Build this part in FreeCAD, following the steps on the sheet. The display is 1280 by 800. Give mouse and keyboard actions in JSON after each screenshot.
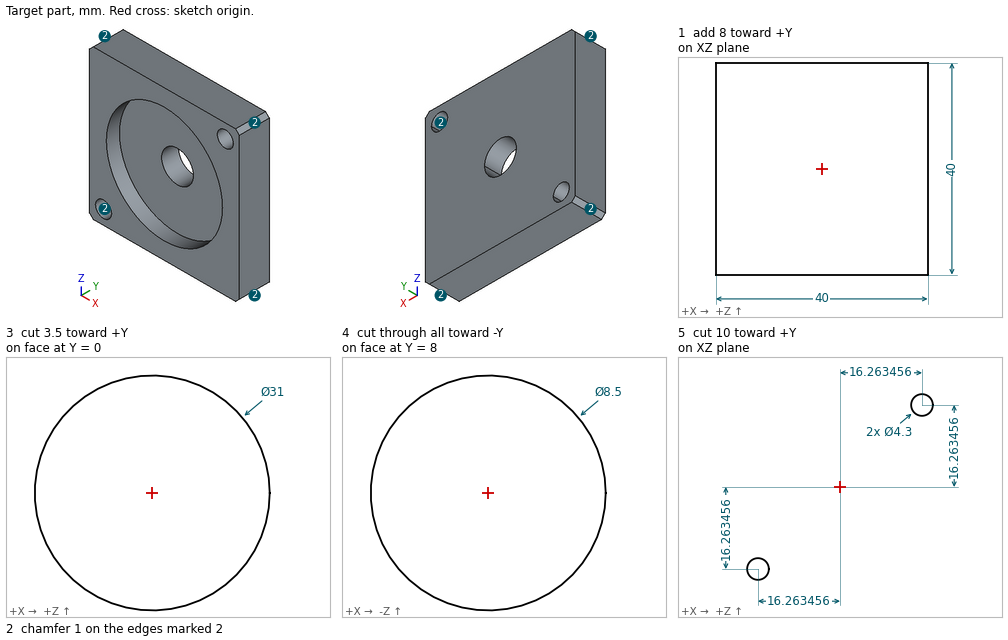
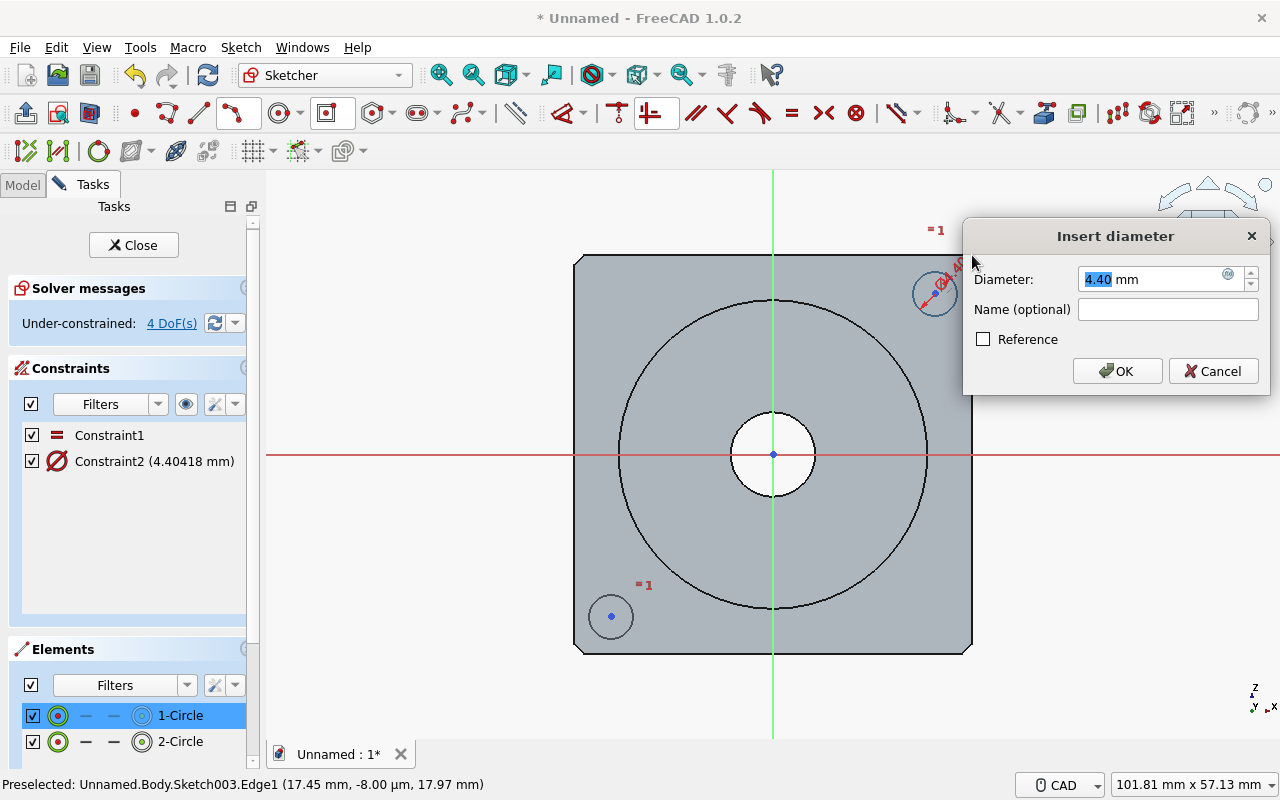
{"action": "type", "text": "4.3"}
{"action": "key", "text": "Return"}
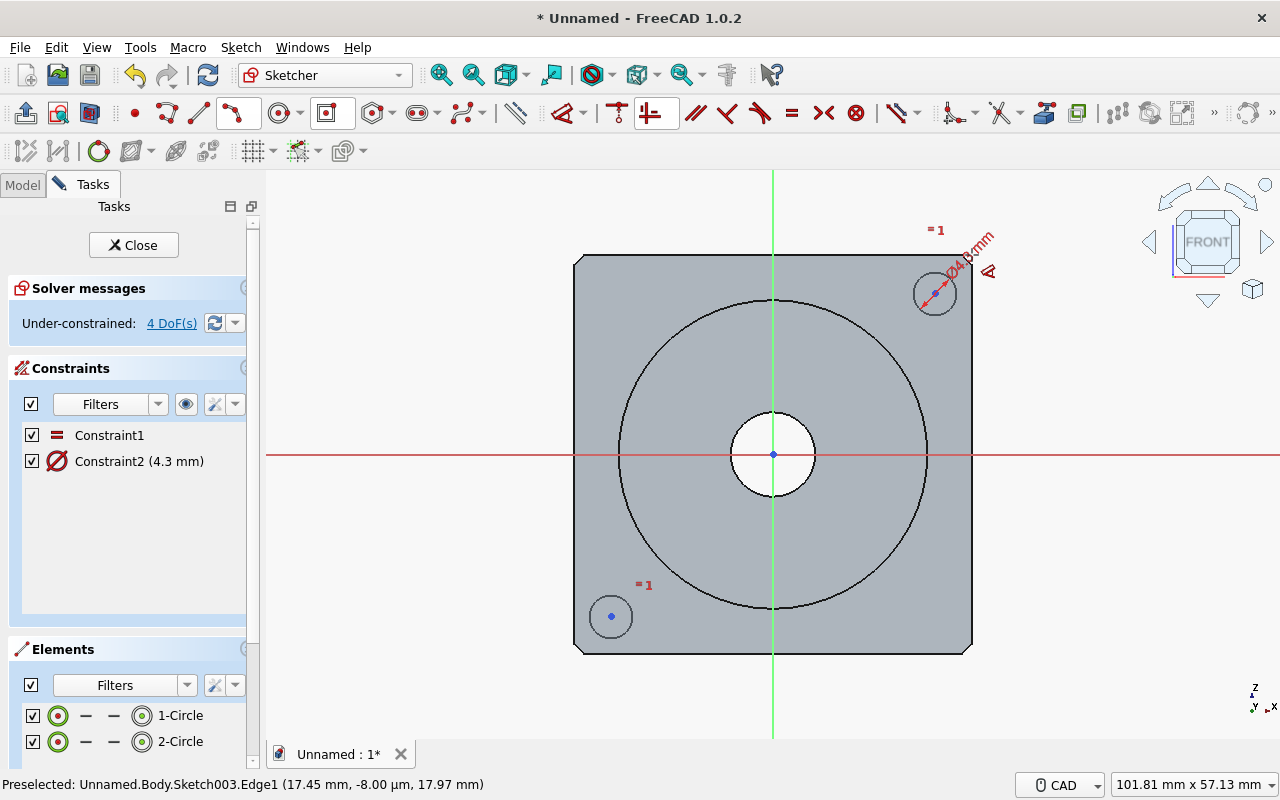
{"action": "left_click", "coordinate": [935, 294]}
{"action": "left_click", "coordinate": [854, 260]}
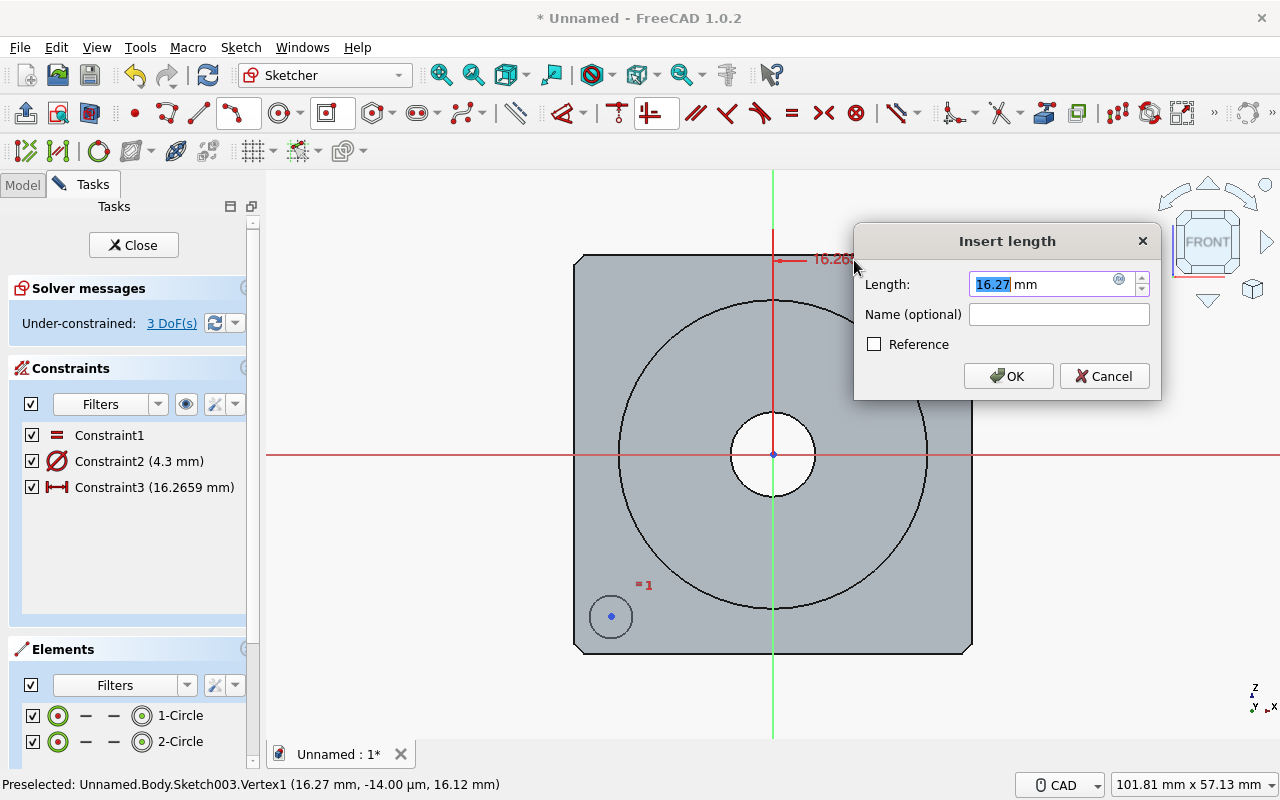
{"action": "type", "text": "16.263456"}
{"action": "key", "text": "Return"}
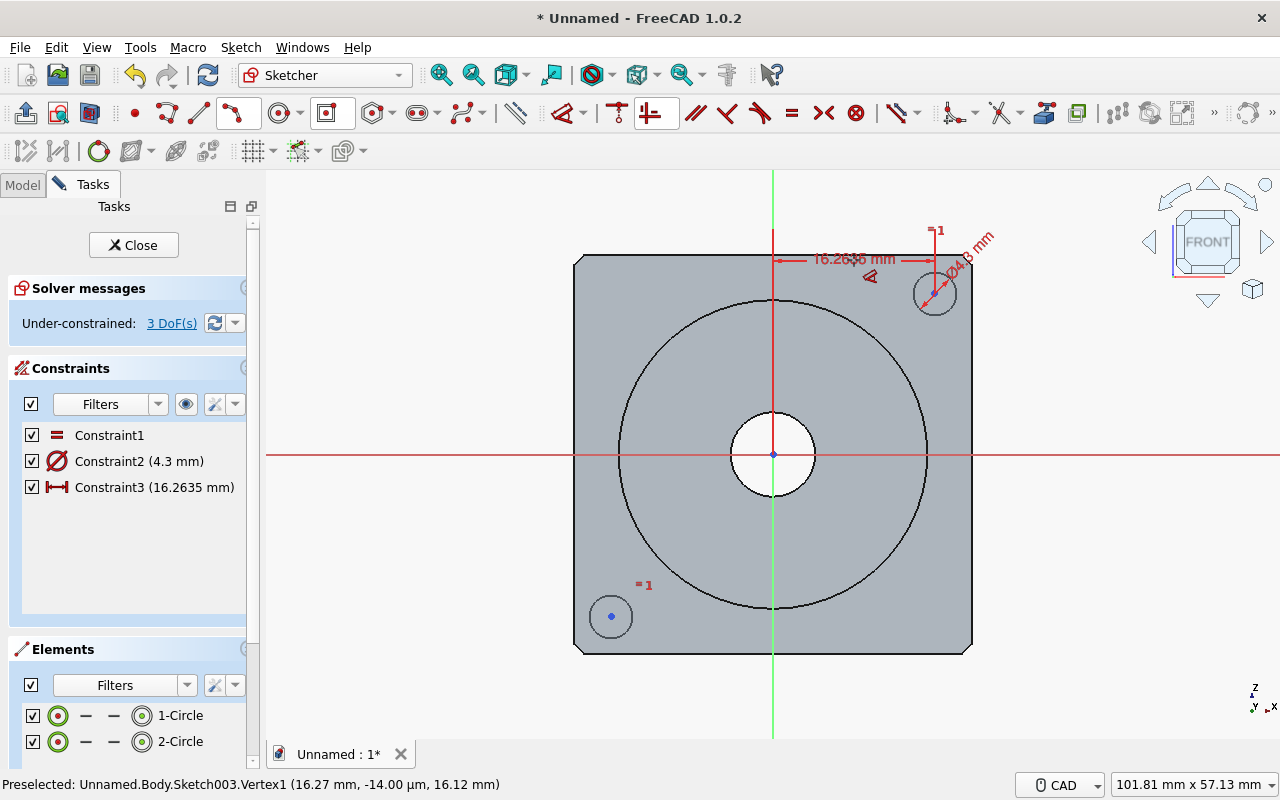
{"action": "left_click", "coordinate": [935, 294]}
{"action": "left_click", "coordinate": [969, 374]}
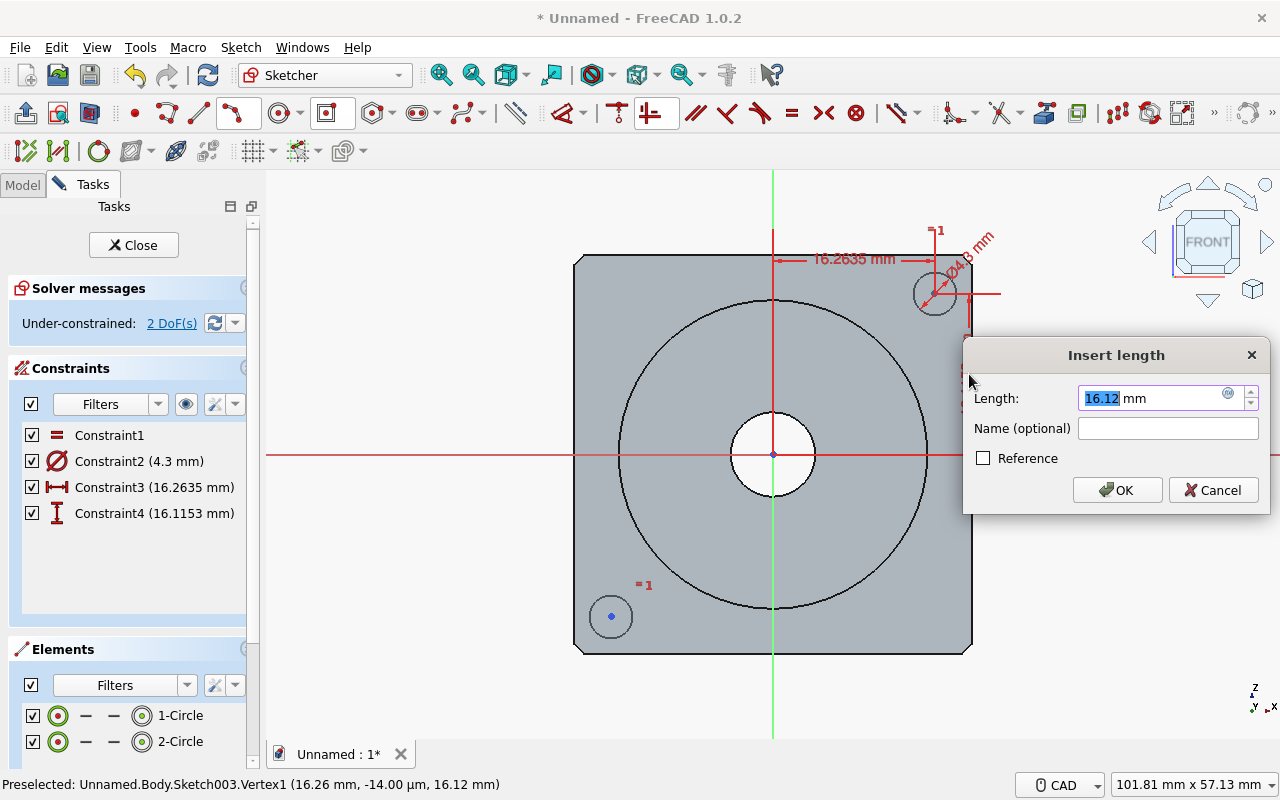
{"action": "type", "text": "16.263456"}
{"action": "key", "text": "Return"}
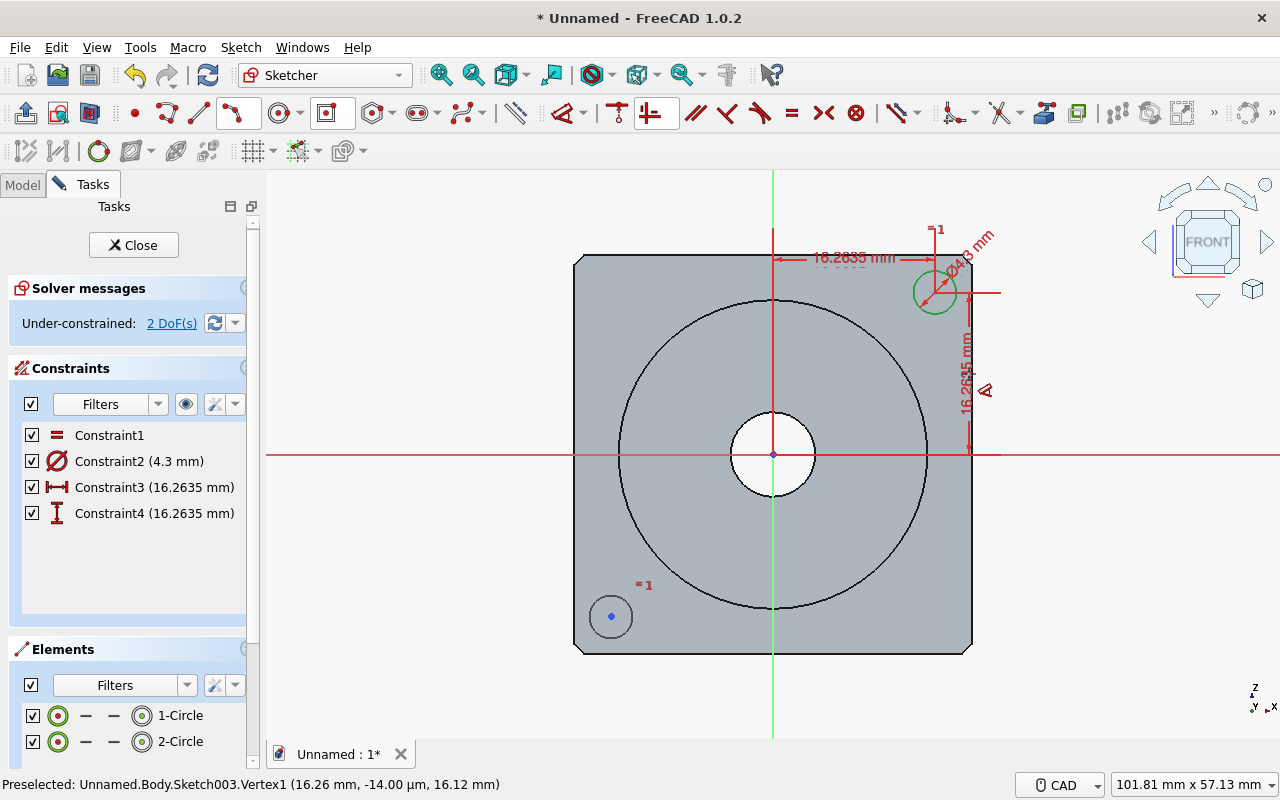
{"action": "left_click", "coordinate": [611, 617]}
{"action": "left_click", "coordinate": [692, 651]}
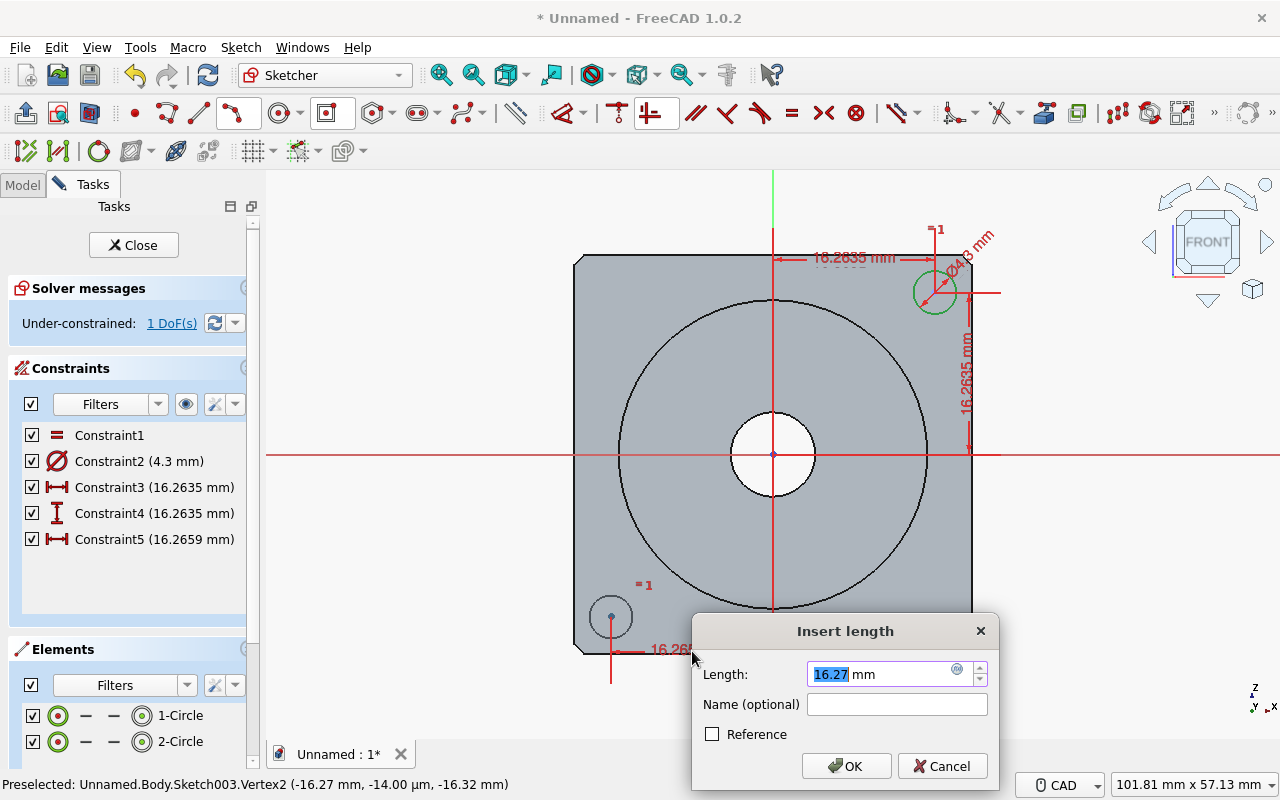
{"action": "type", "text": "16.263456"}
{"action": "key", "text": "Return"}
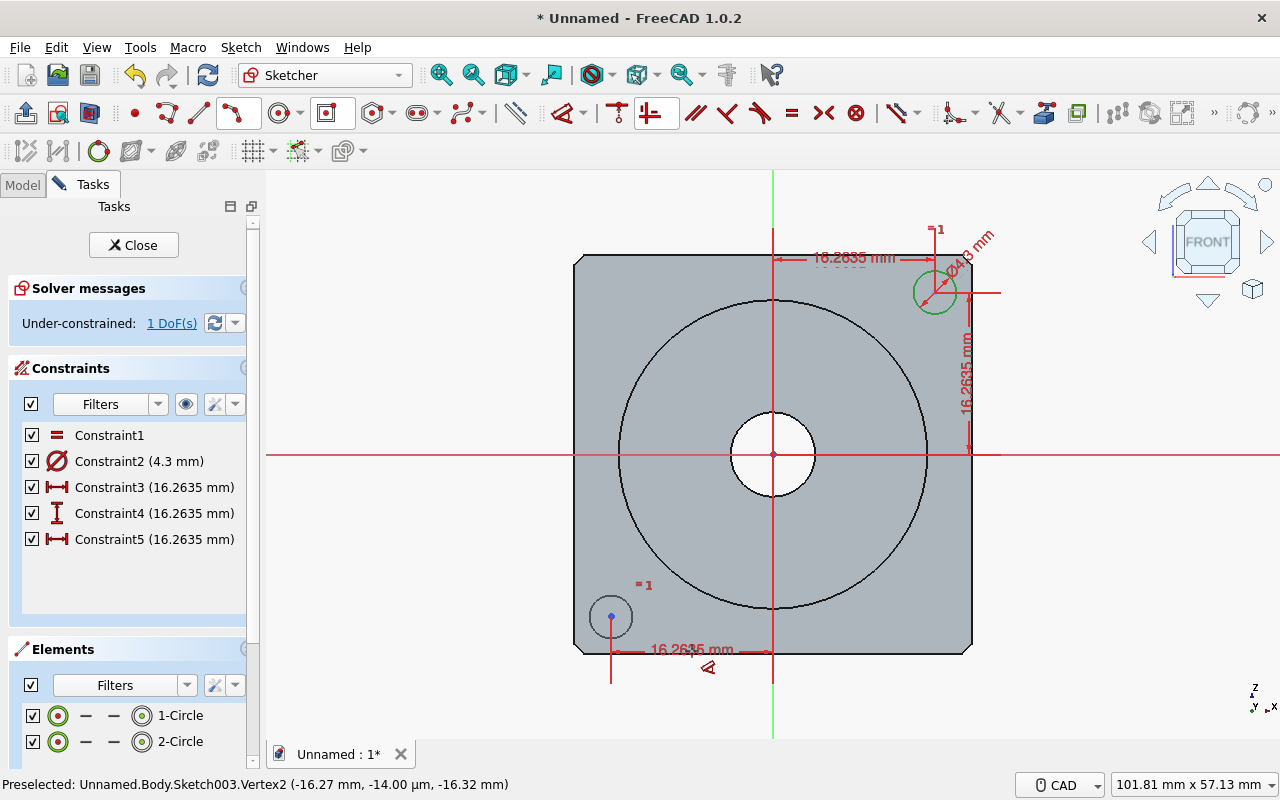
{"action": "left_click", "coordinate": [611, 617]}
{"action": "left_click", "coordinate": [577, 536]}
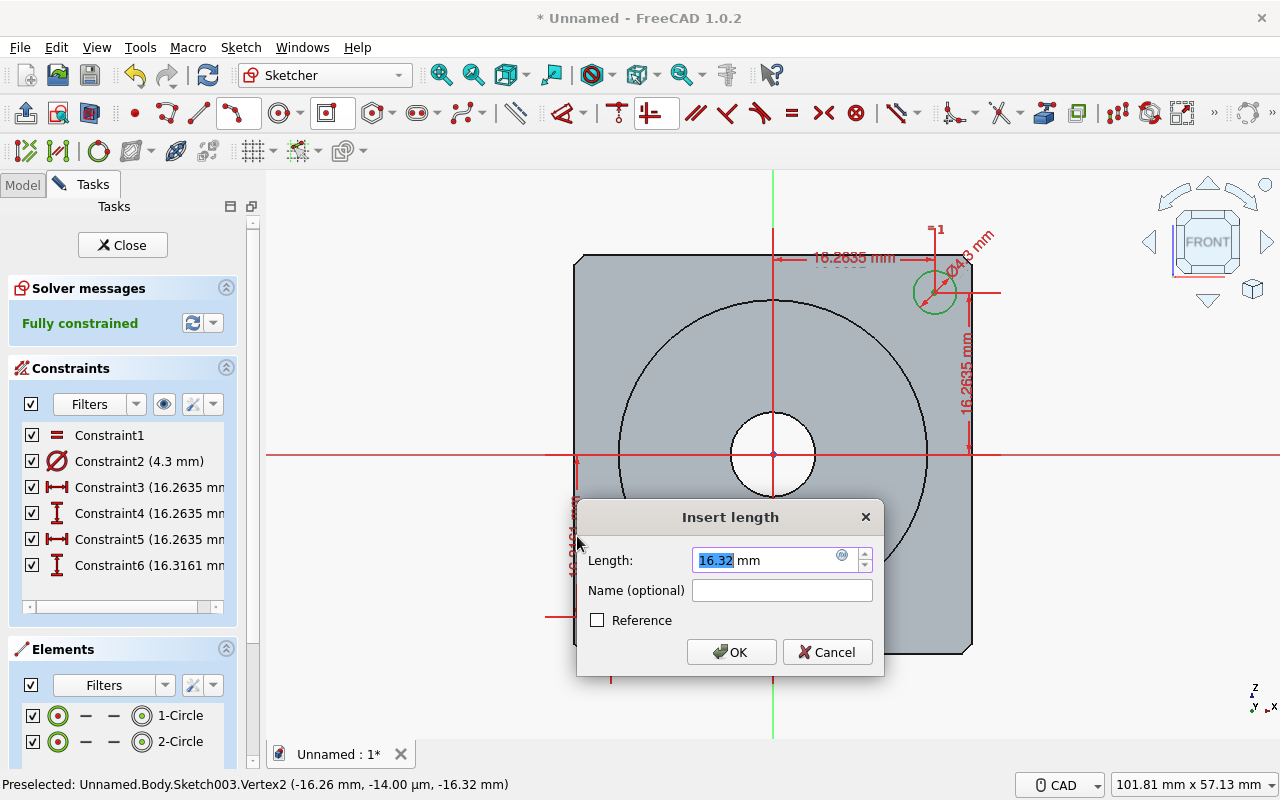
{"action": "type", "text": "16.263456"}
{"action": "key", "text": "Return"}
{"action": "key", "text": "Escape"}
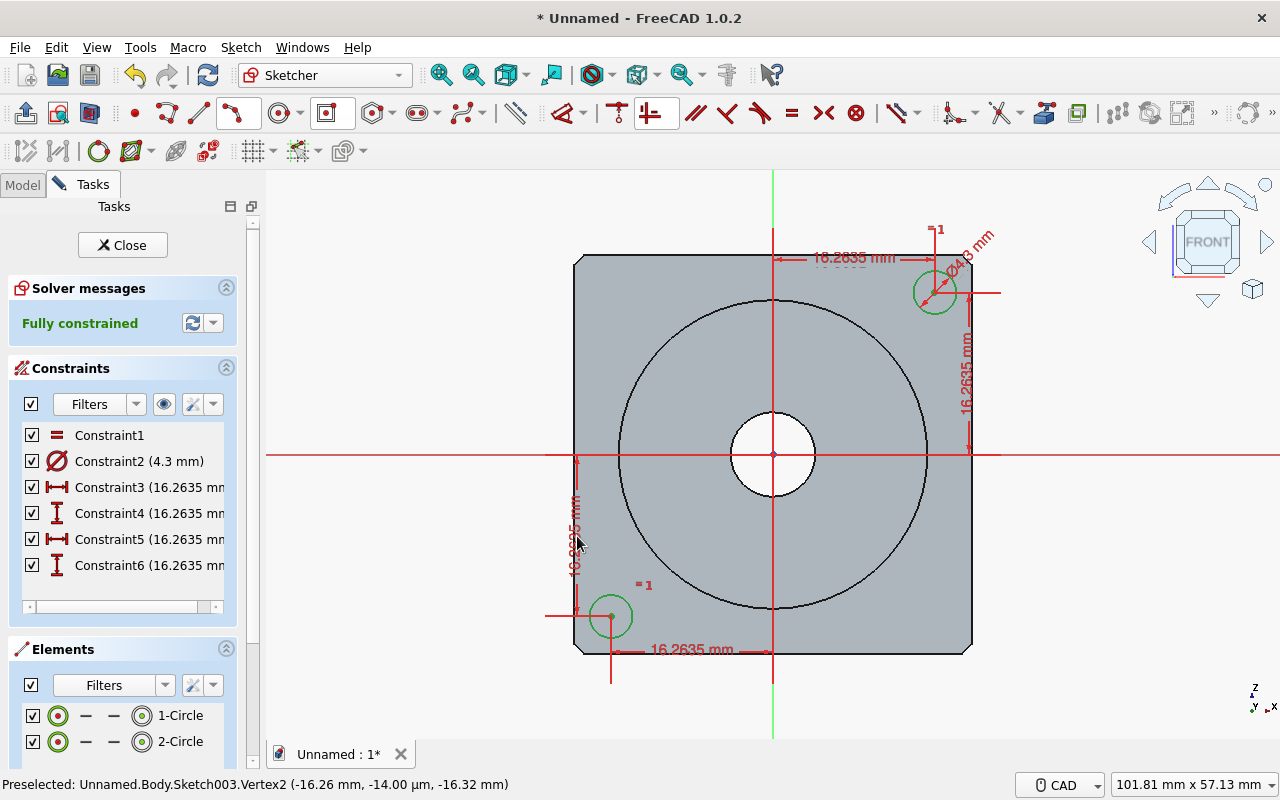
{"action": "left_click", "coordinate": [123, 245]}